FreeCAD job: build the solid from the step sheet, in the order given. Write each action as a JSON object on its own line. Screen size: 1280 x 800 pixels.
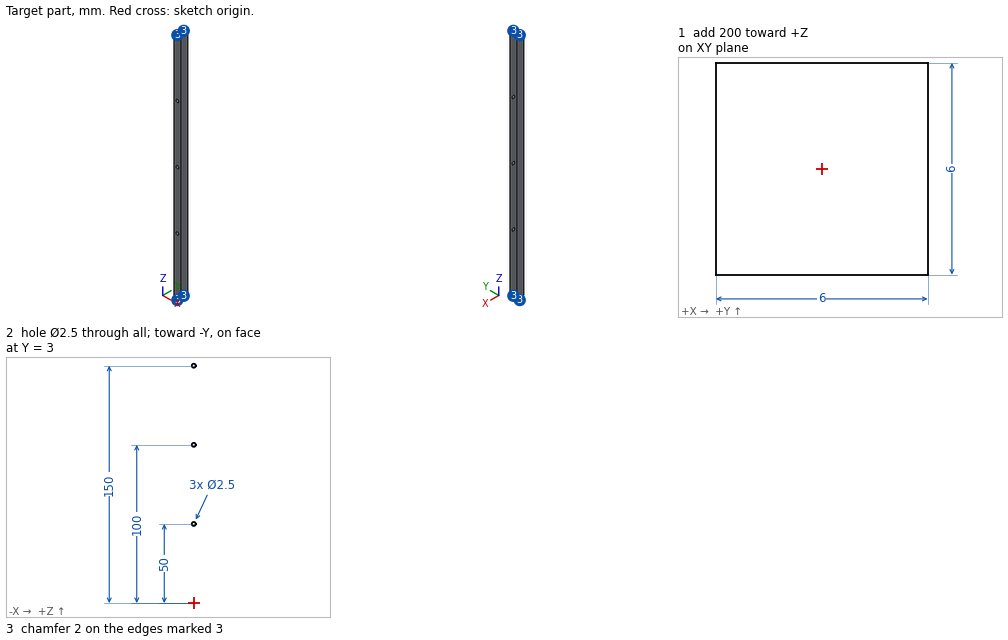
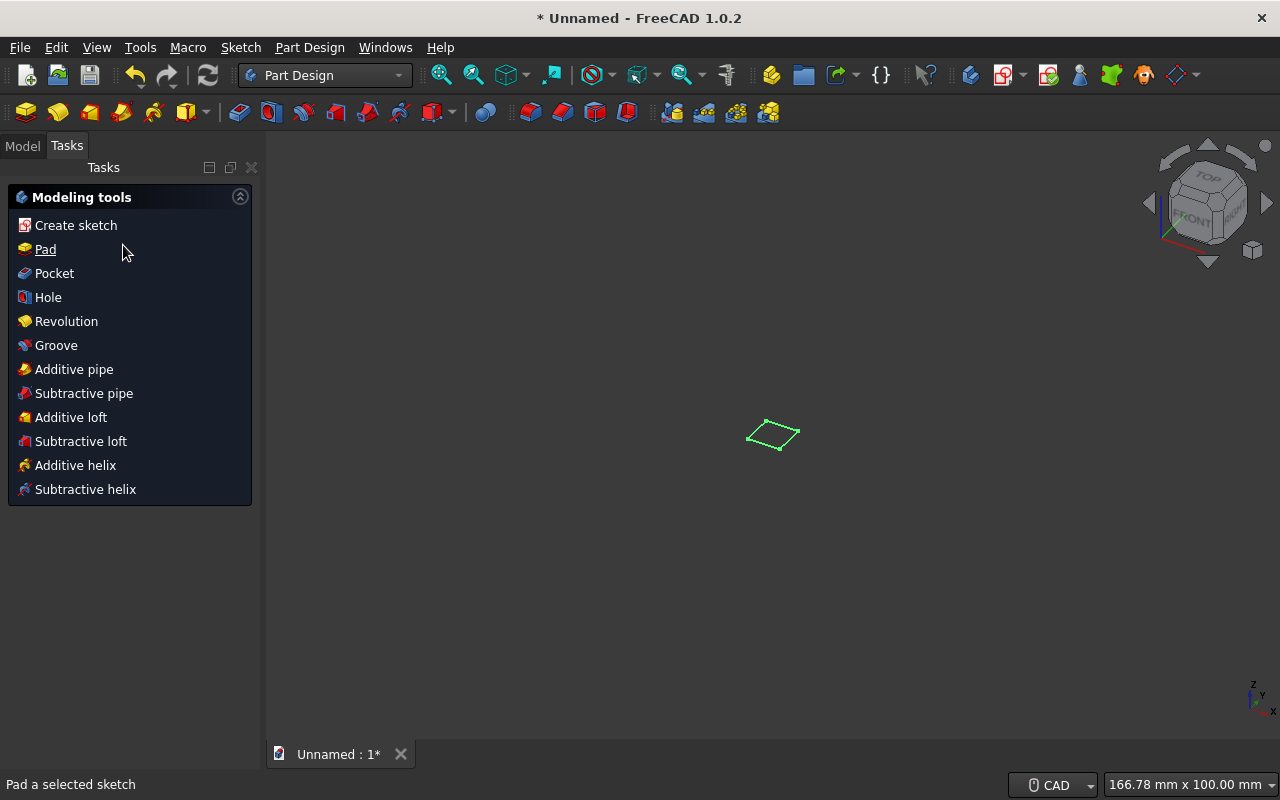
{"action": "left_click", "coordinate": [26, 112]}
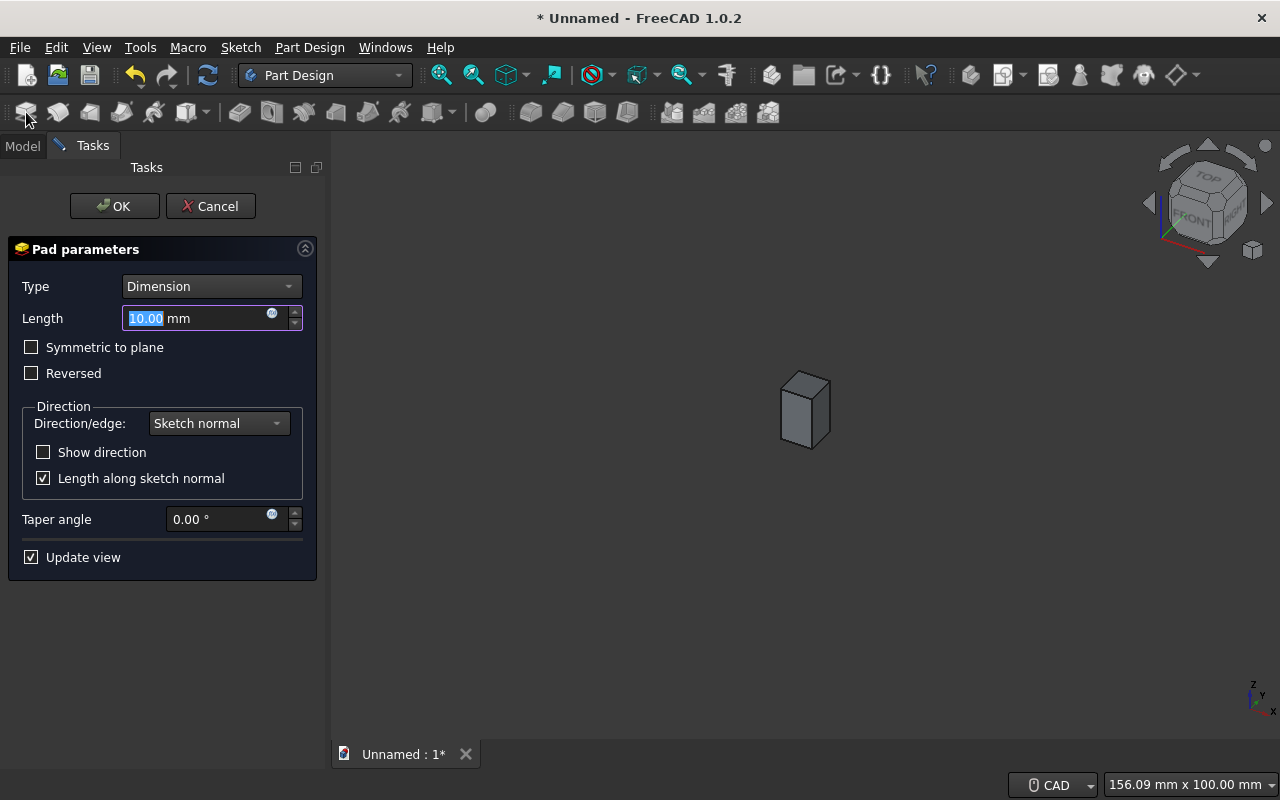
{"action": "type", "text": "200"}
{"action": "key", "text": "Tab"}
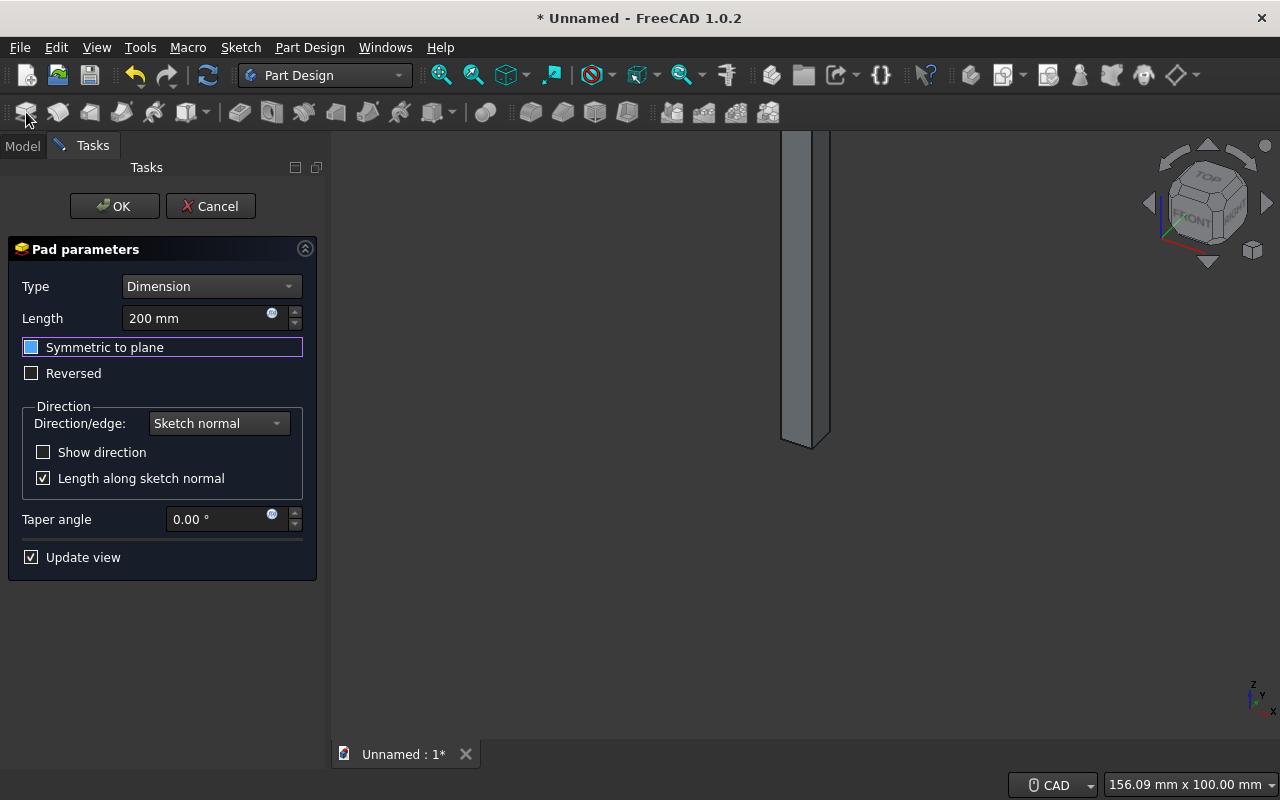
{"action": "left_click", "coordinate": [115, 206]}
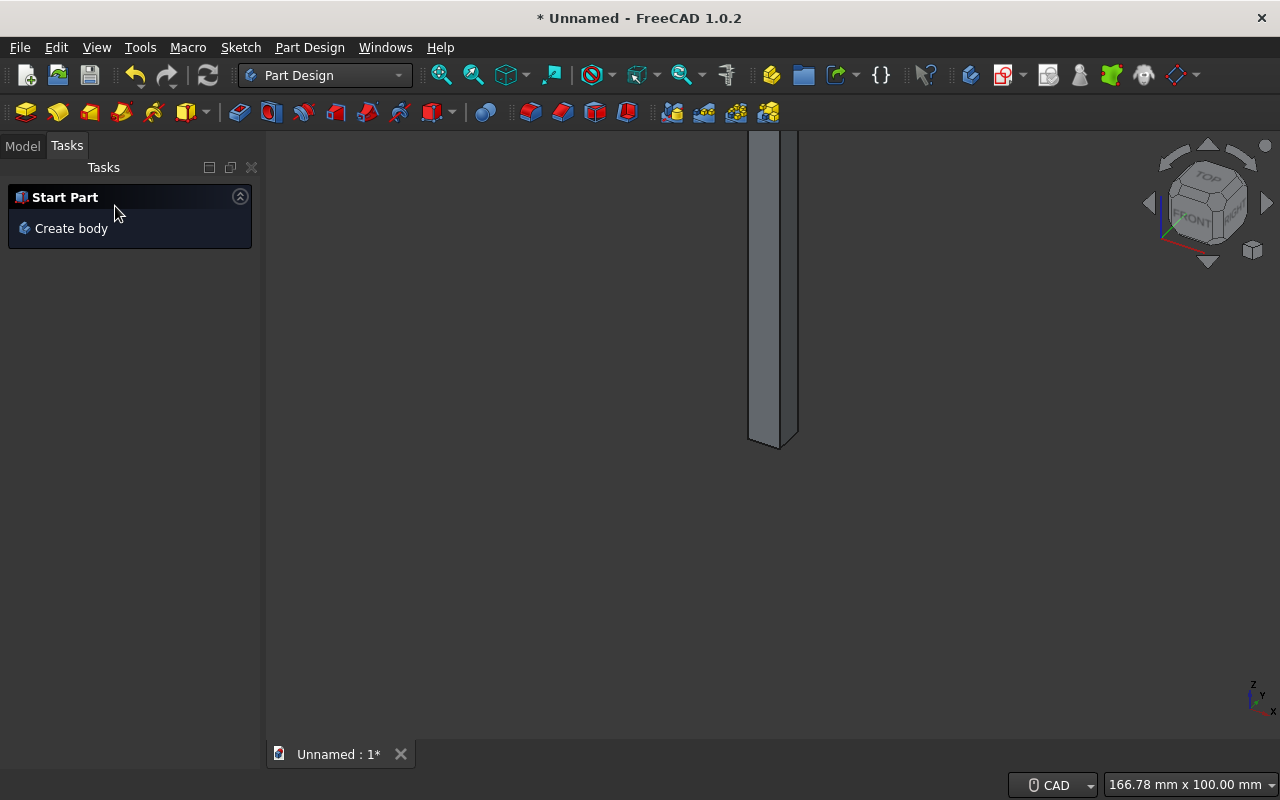
{"action": "left_click", "coordinate": [442, 76]}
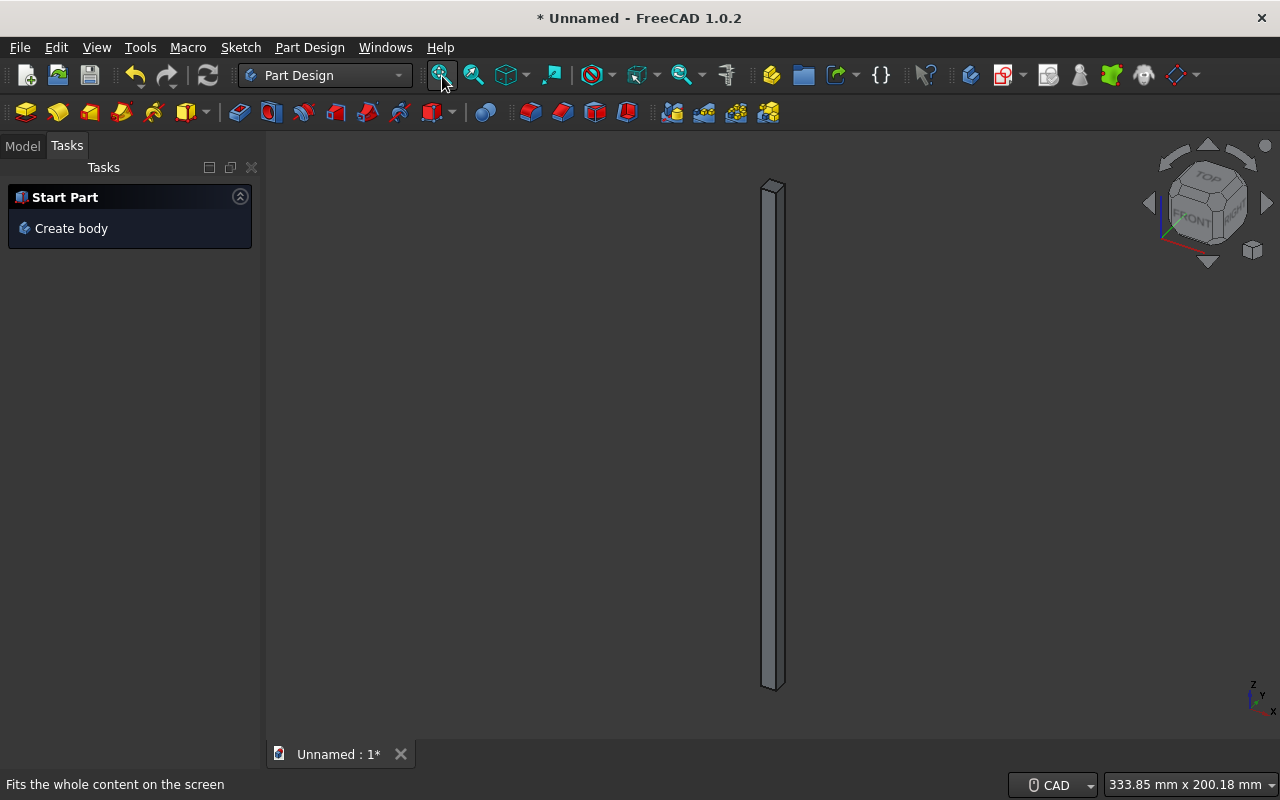
{"action": "key", "text": "4"}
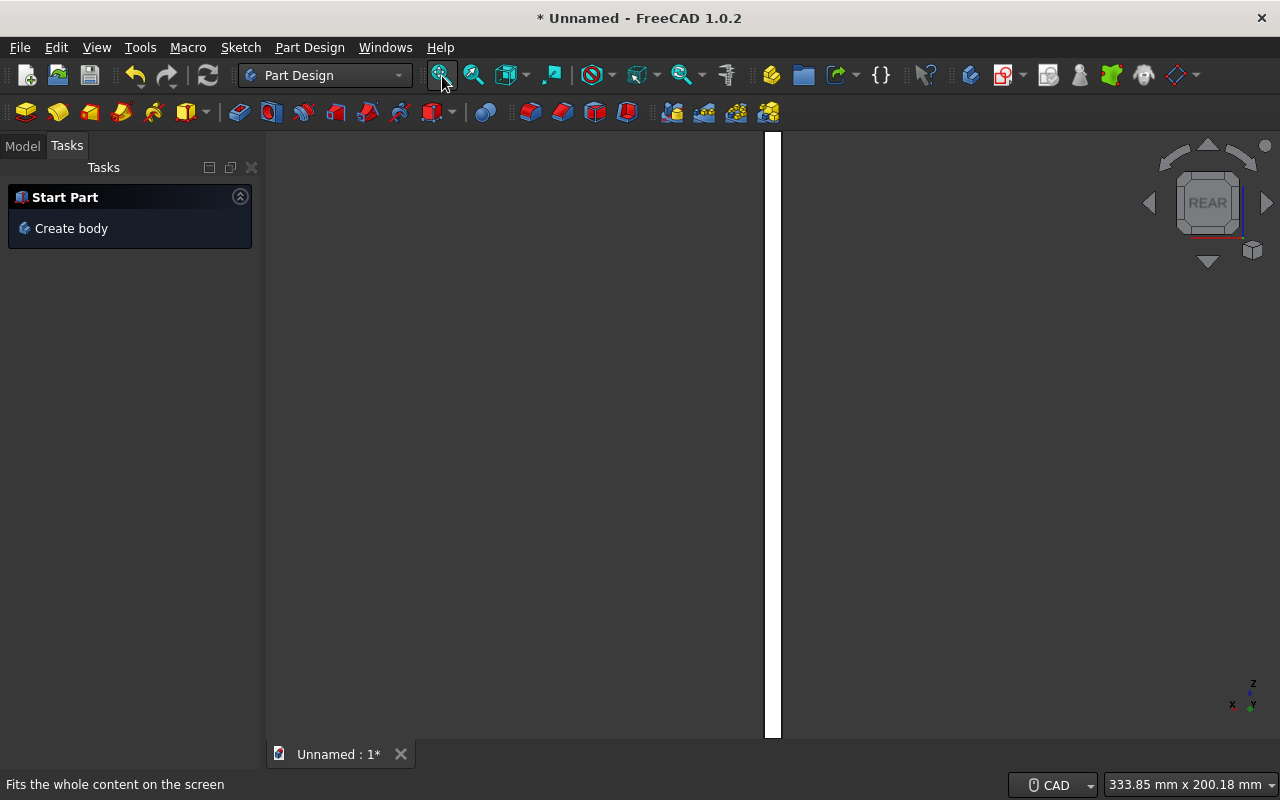
{"action": "left_click", "coordinate": [442, 76]}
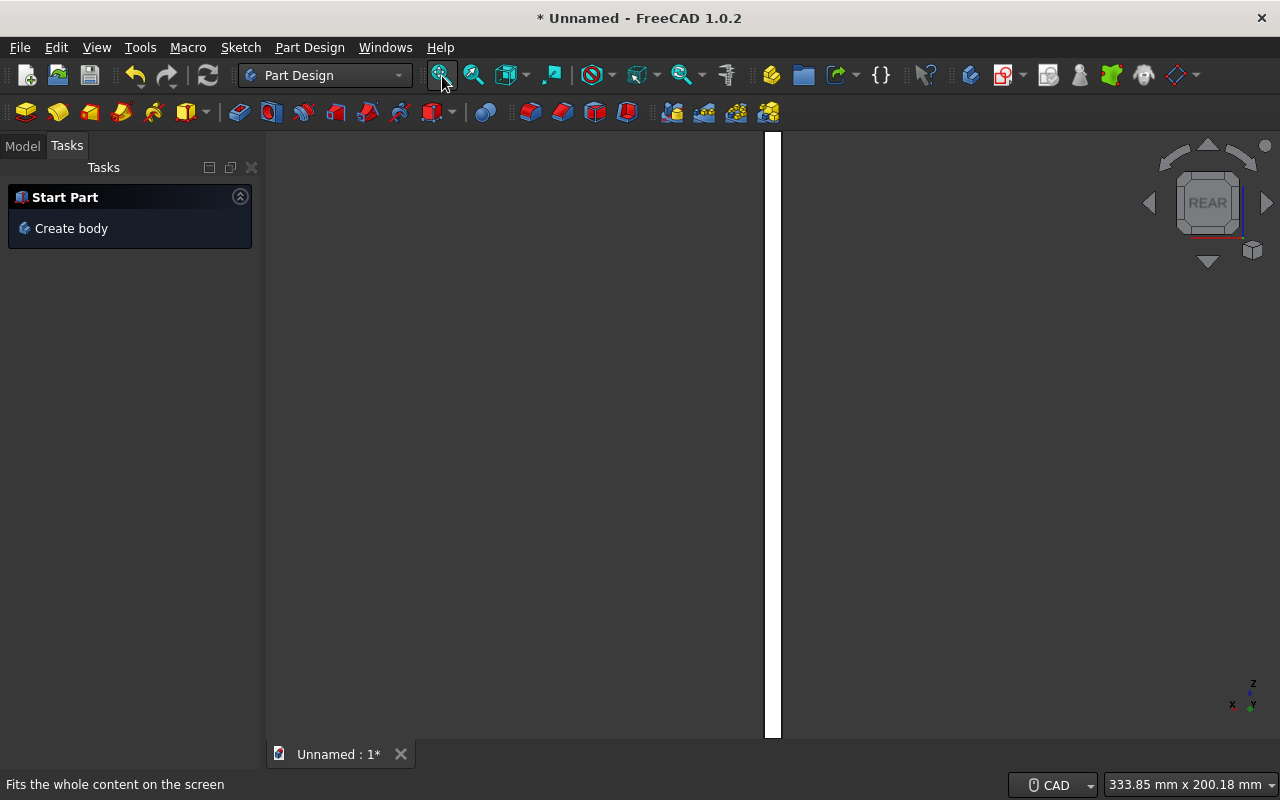
{"action": "left_click", "coordinate": [773, 174]}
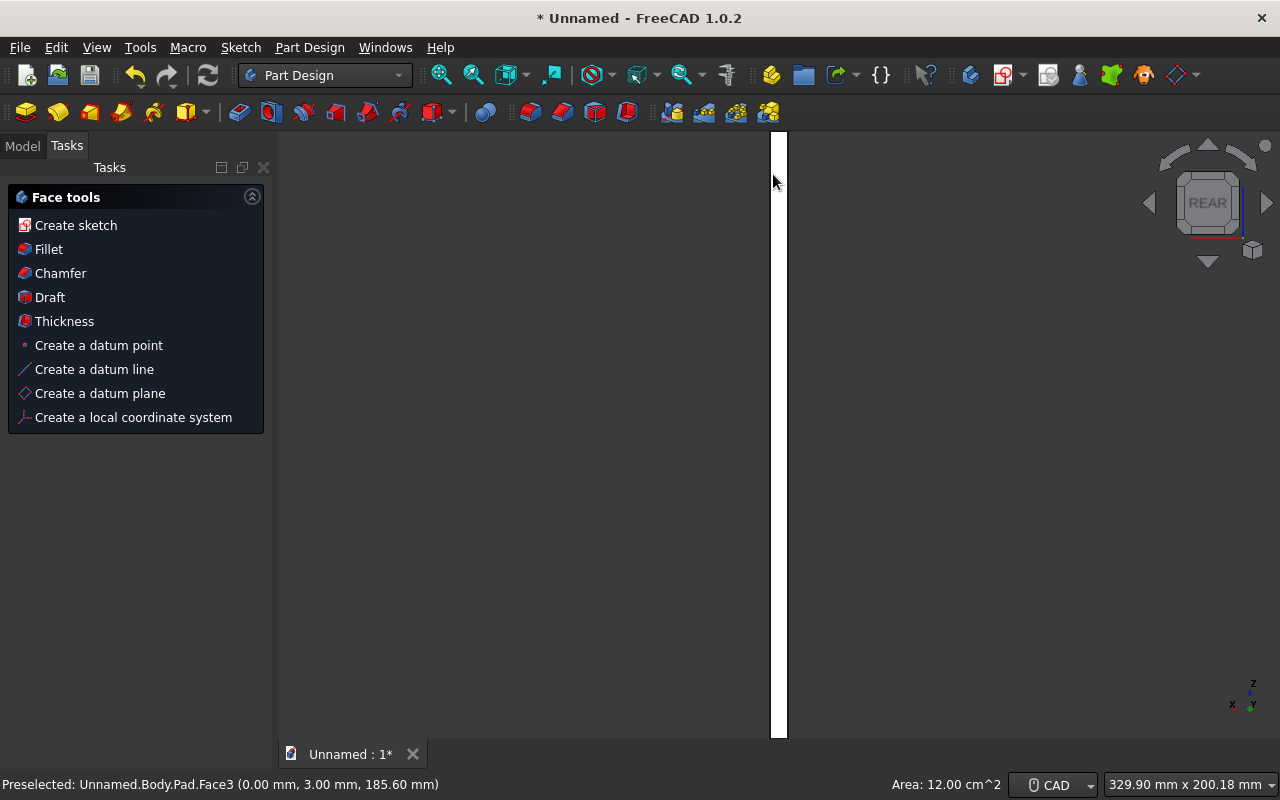
{"action": "left_click", "coordinate": [1004, 76]}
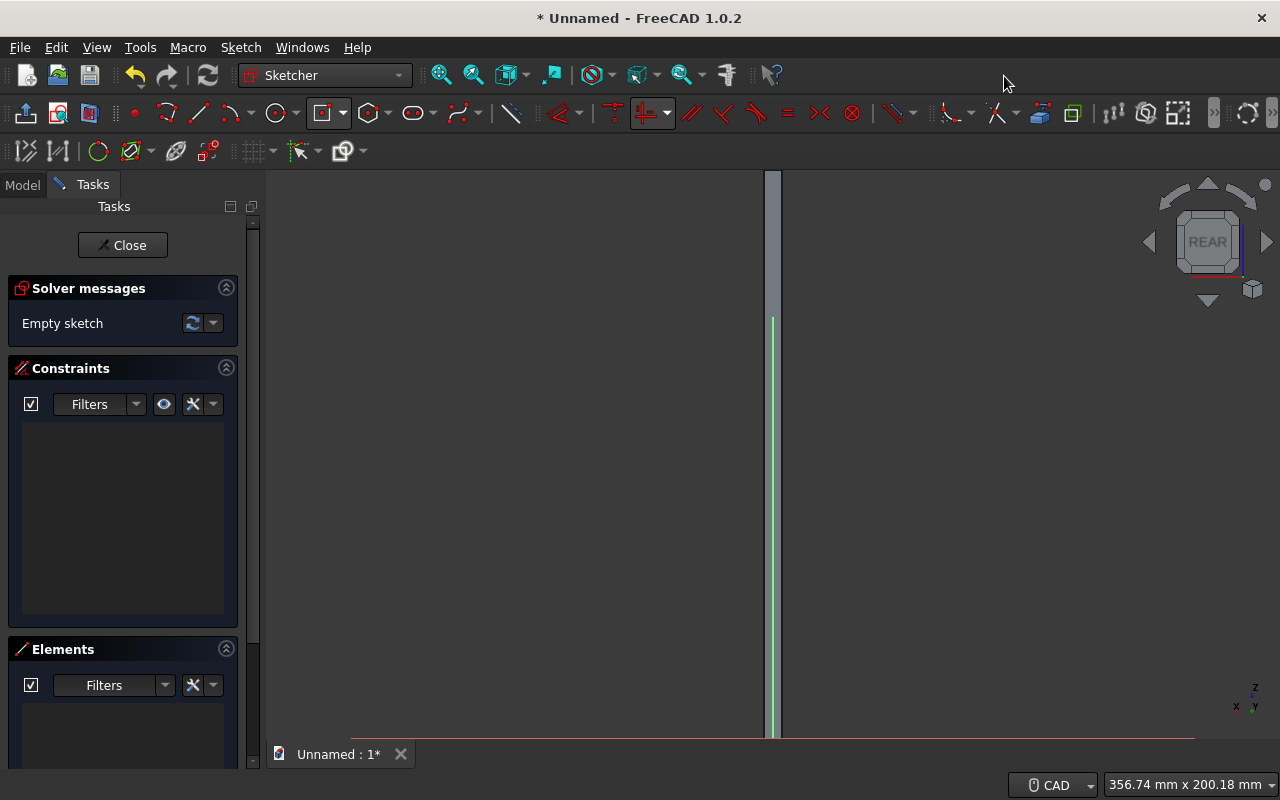
{"action": "scroll", "coordinate": [395, 198], "scroll_direction": "down", "scroll_amount": 1}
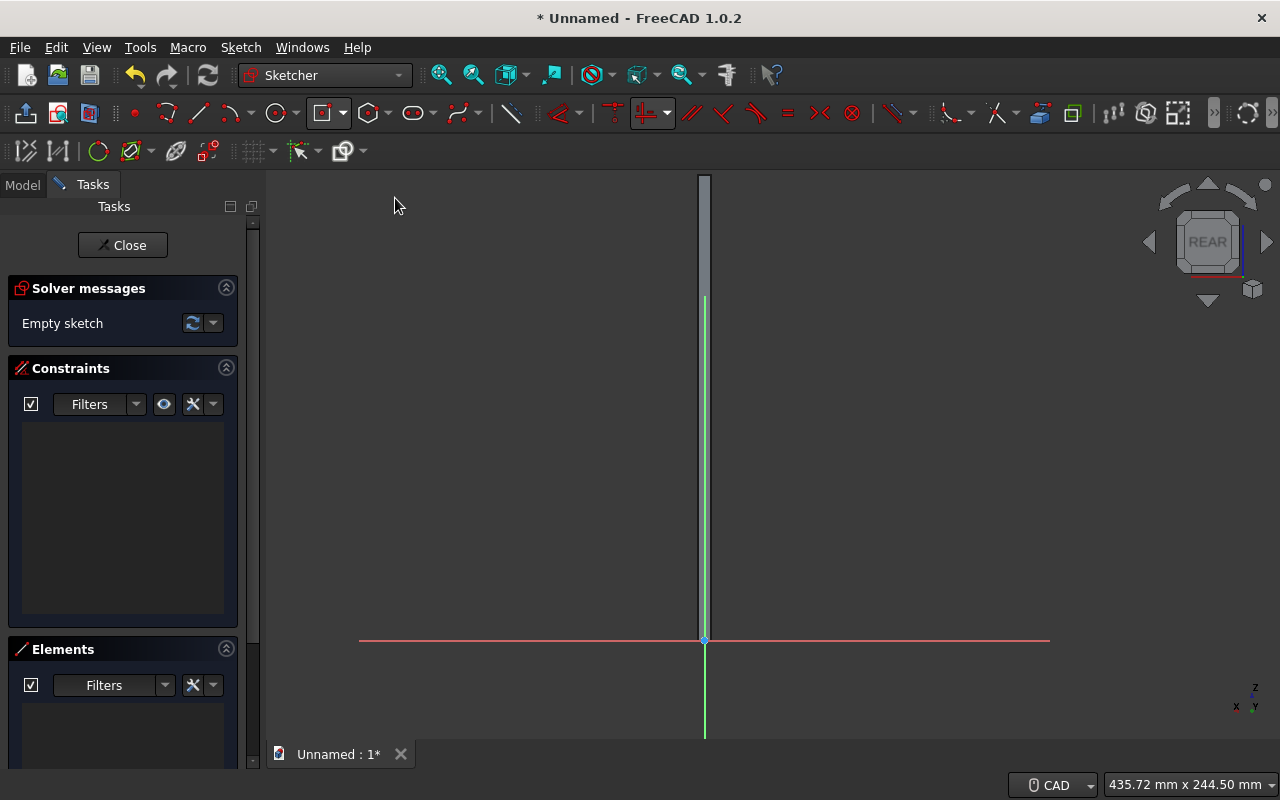
{"action": "left_click", "coordinate": [276, 114]}